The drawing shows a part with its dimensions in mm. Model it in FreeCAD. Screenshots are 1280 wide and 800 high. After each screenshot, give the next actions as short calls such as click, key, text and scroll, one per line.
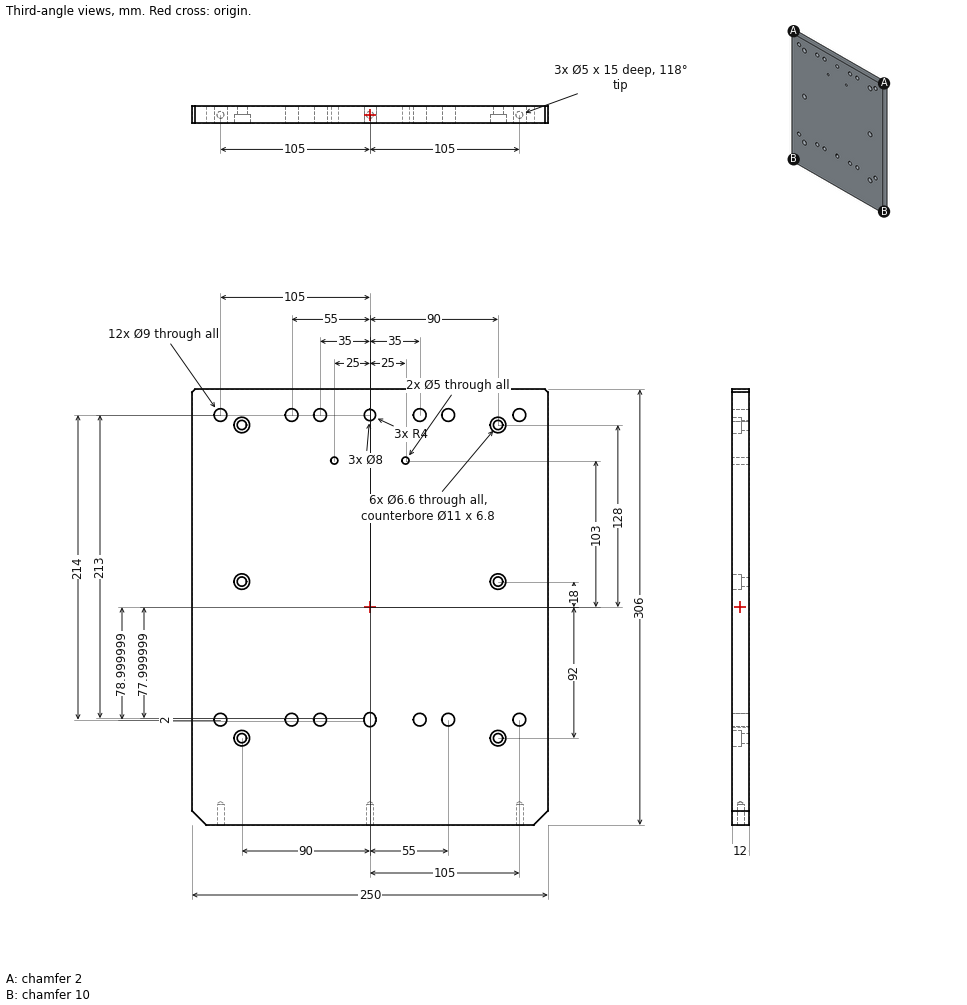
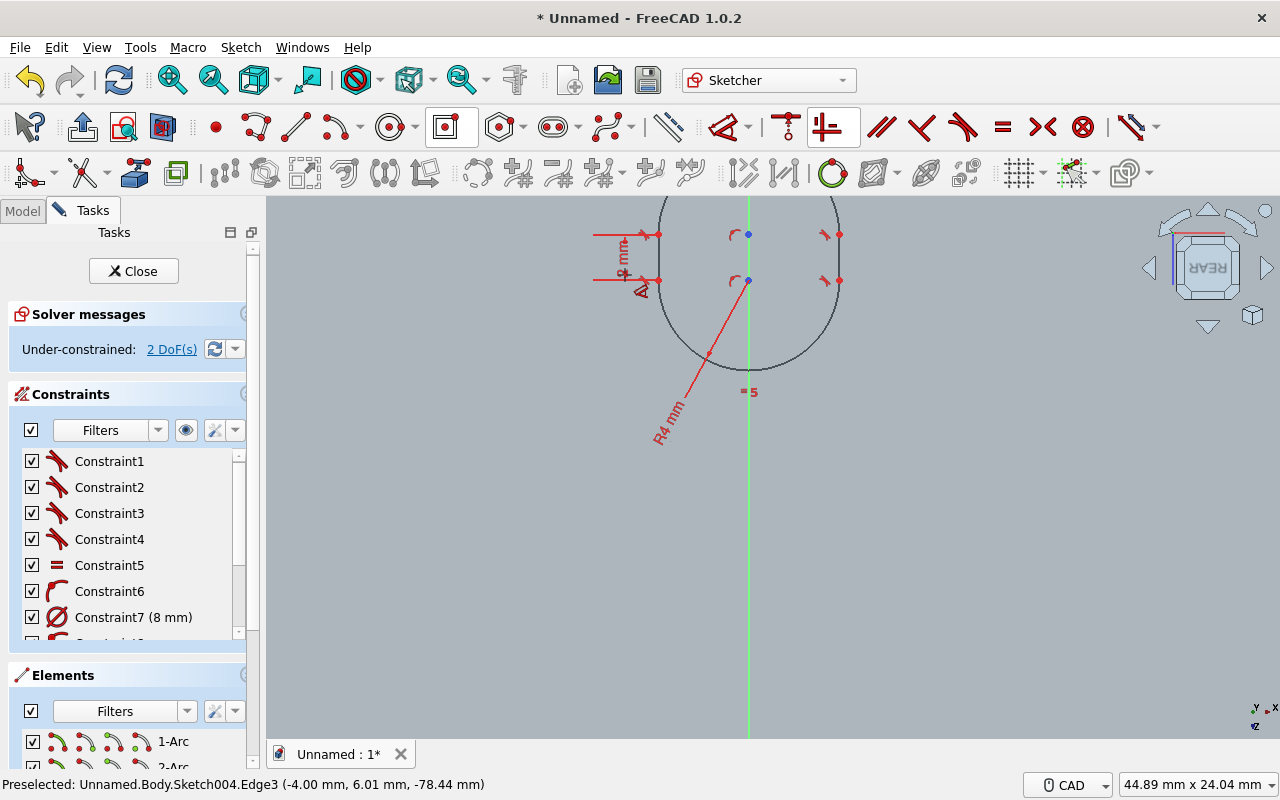
scroll(701, 291, down, 13)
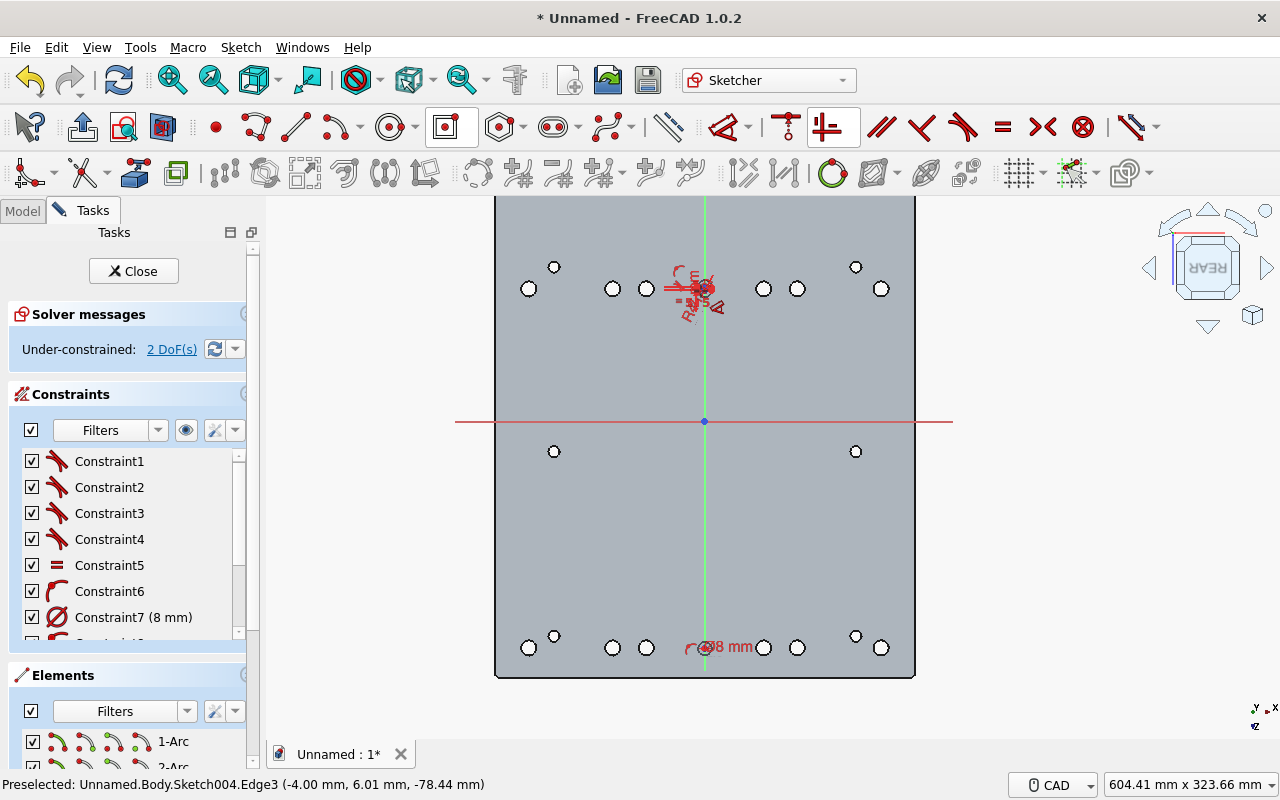
scroll(698, 290, up, 7)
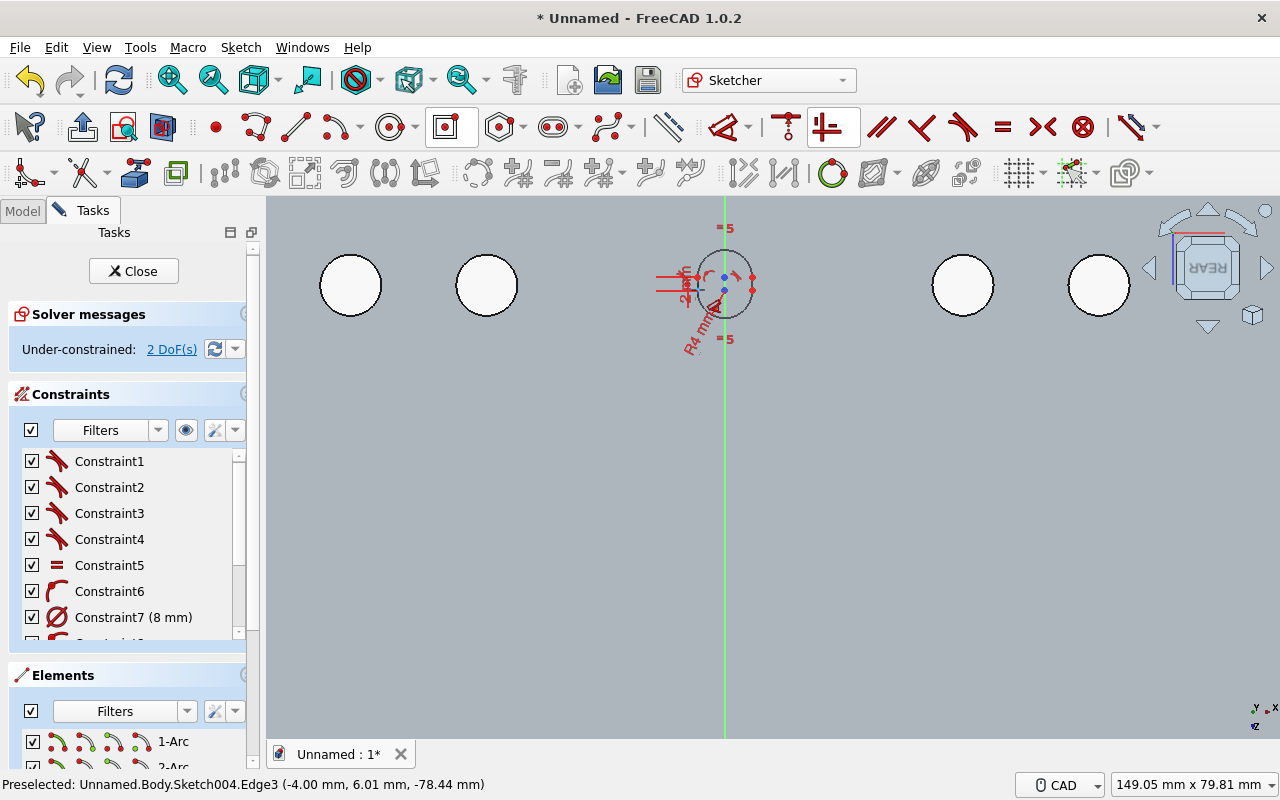
click(698, 291)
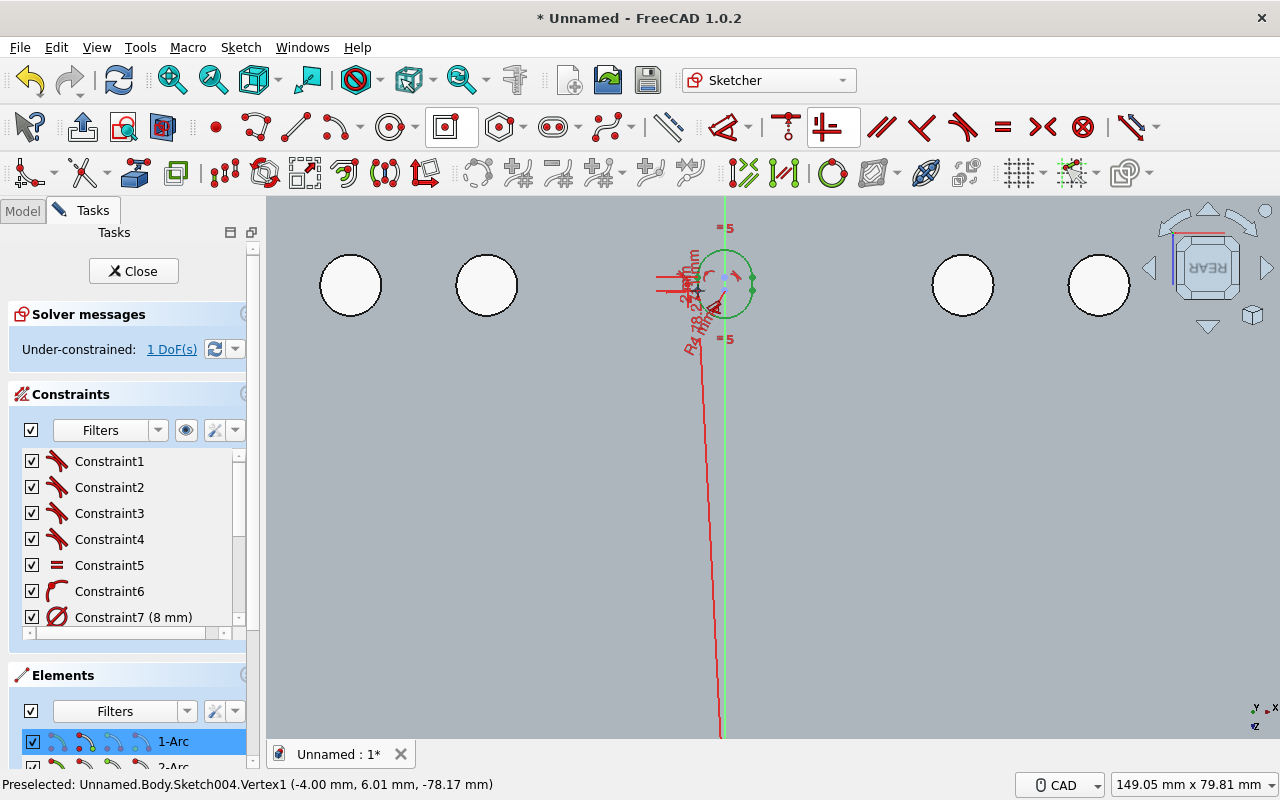
scroll(698, 290, down, 7)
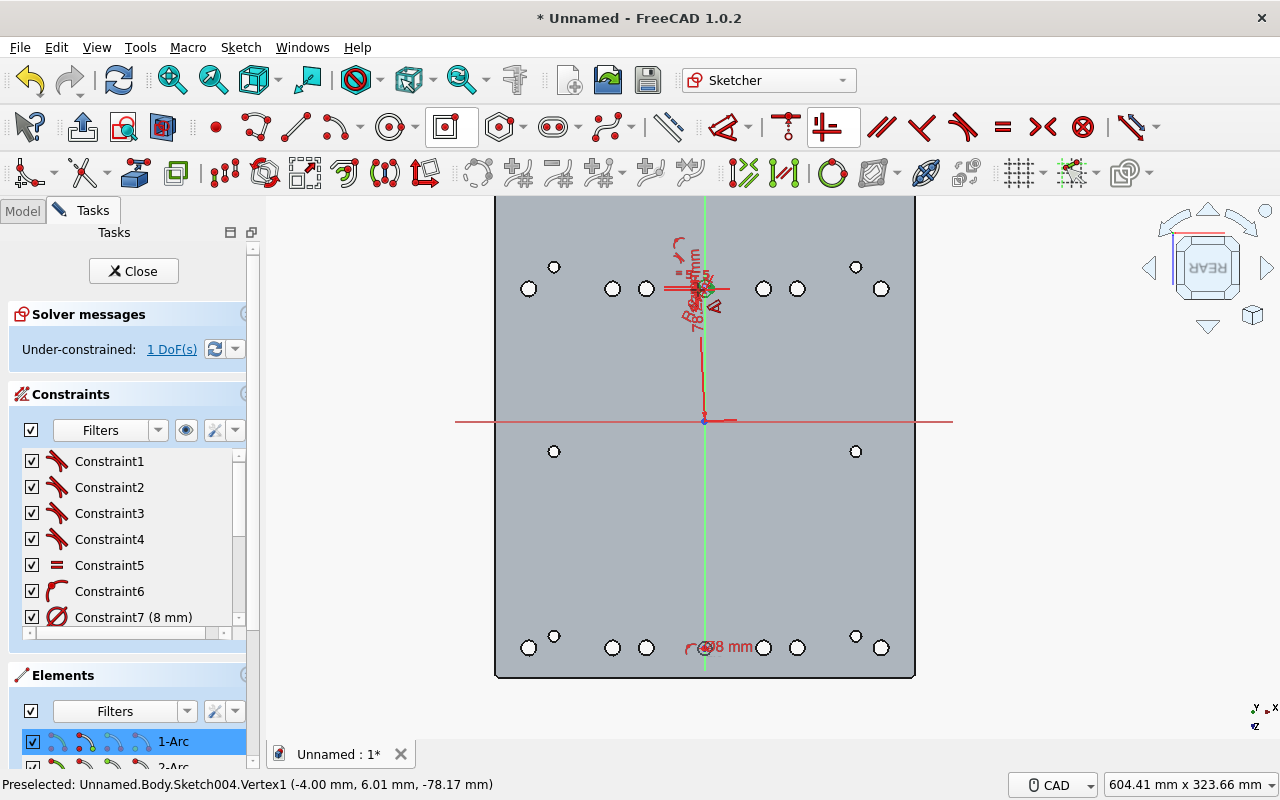
click(705, 649)
click(664, 470)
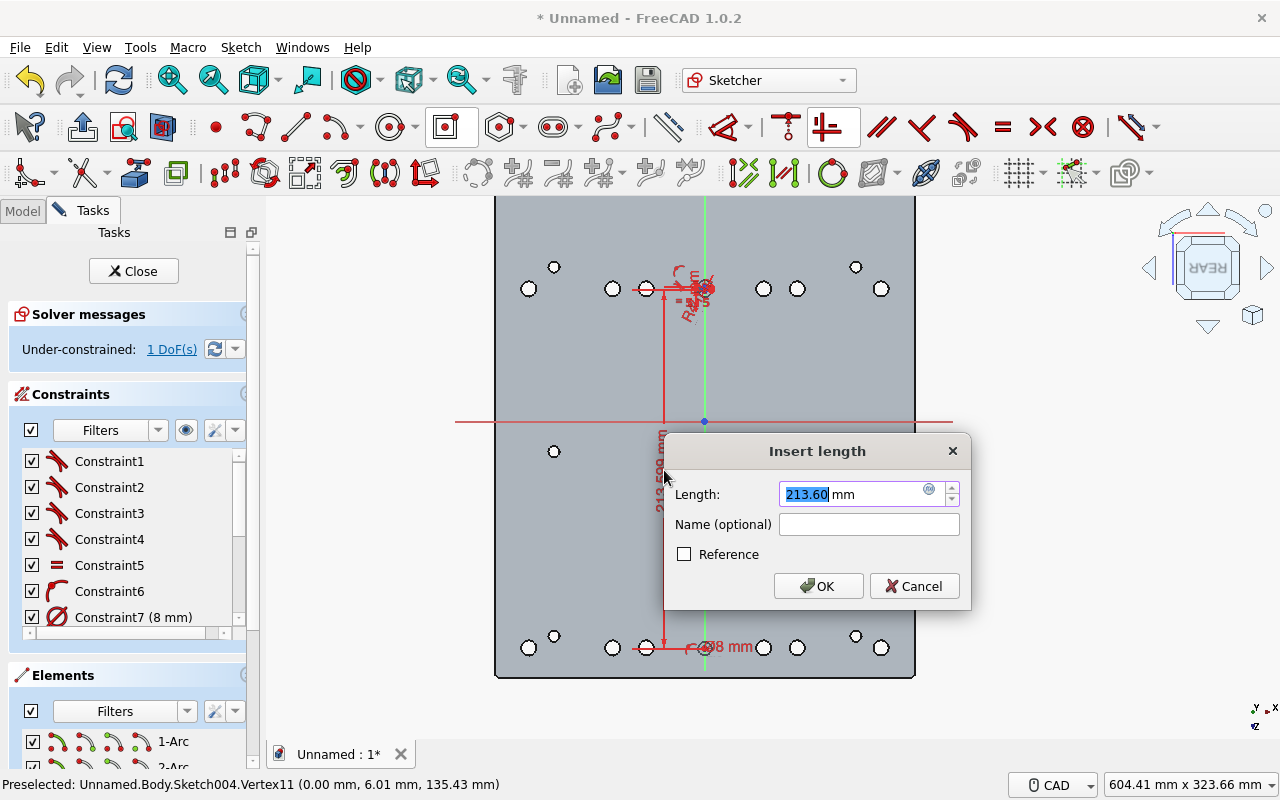
text(213)
key(Return)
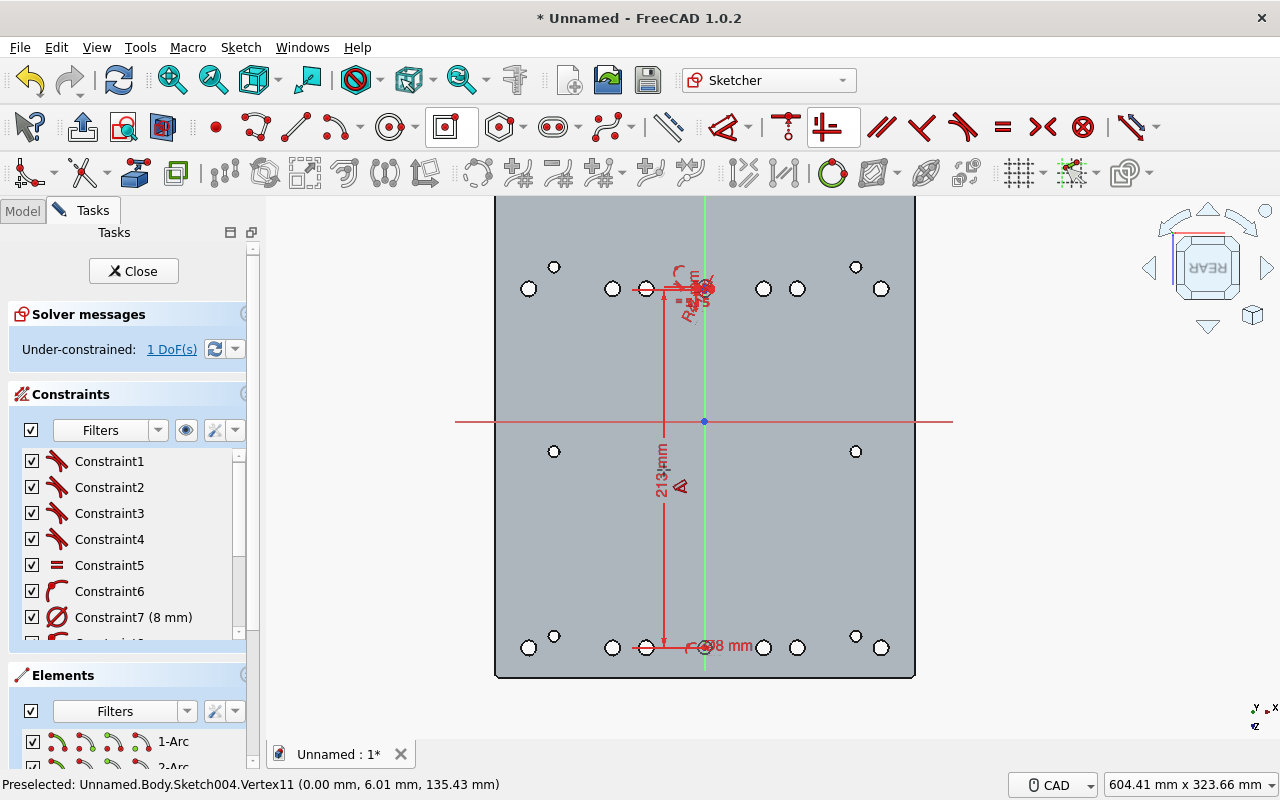
scroll(698, 290, up, 7)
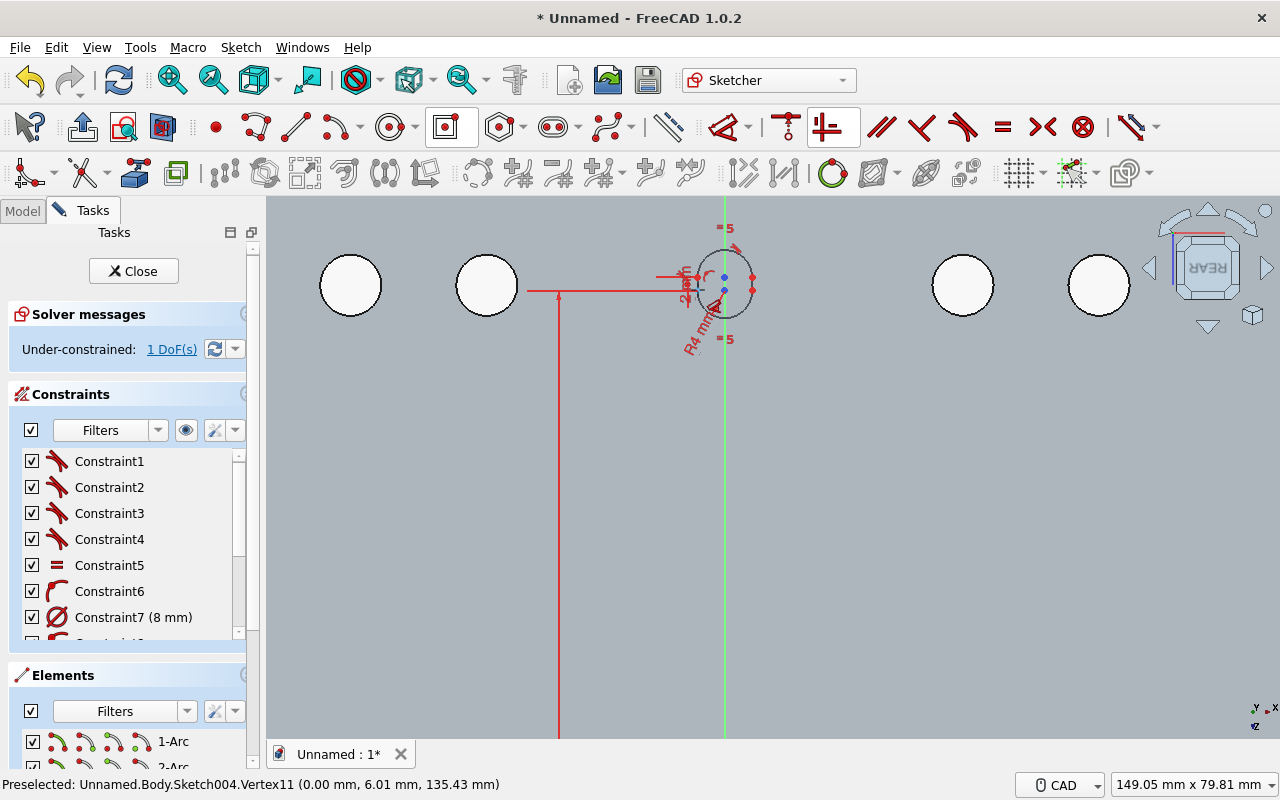
click(698, 291)
click(664, 501)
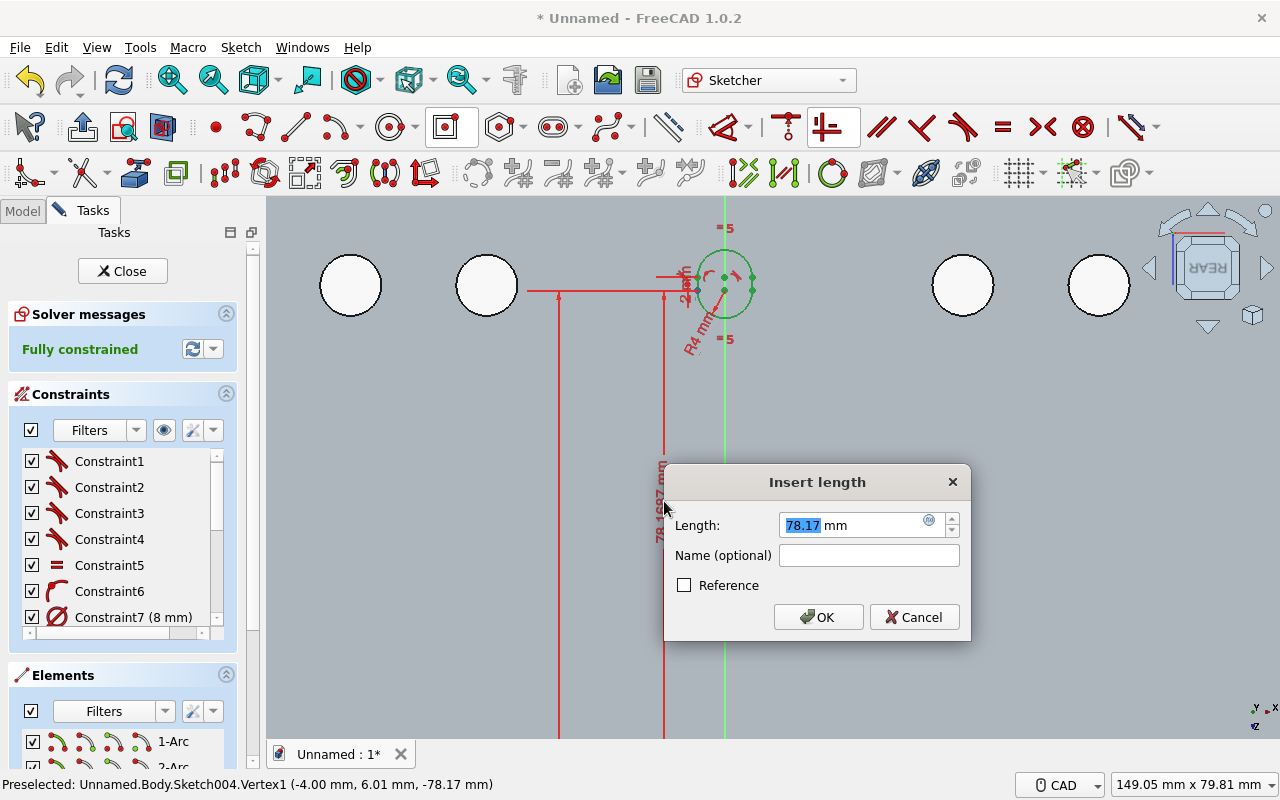
text(77.999999)
key(Return)
key(Escape)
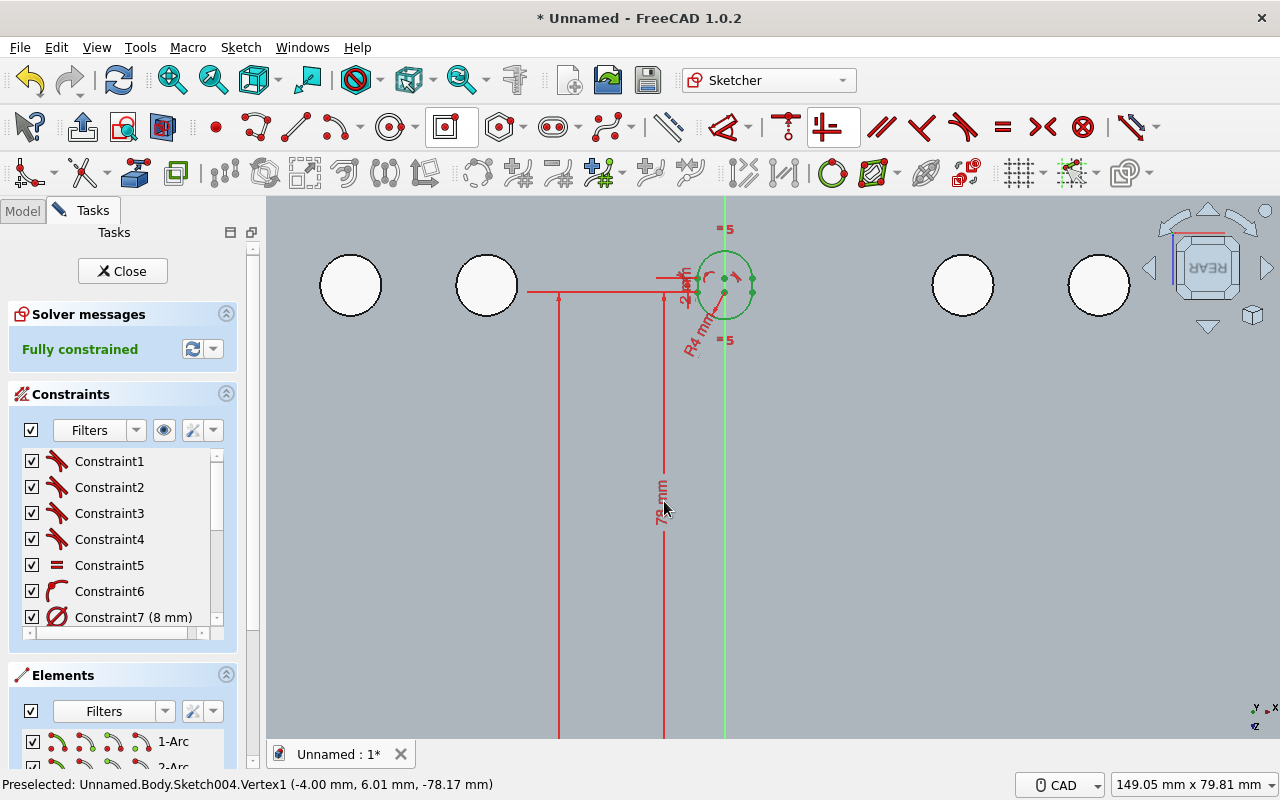
click(123, 271)